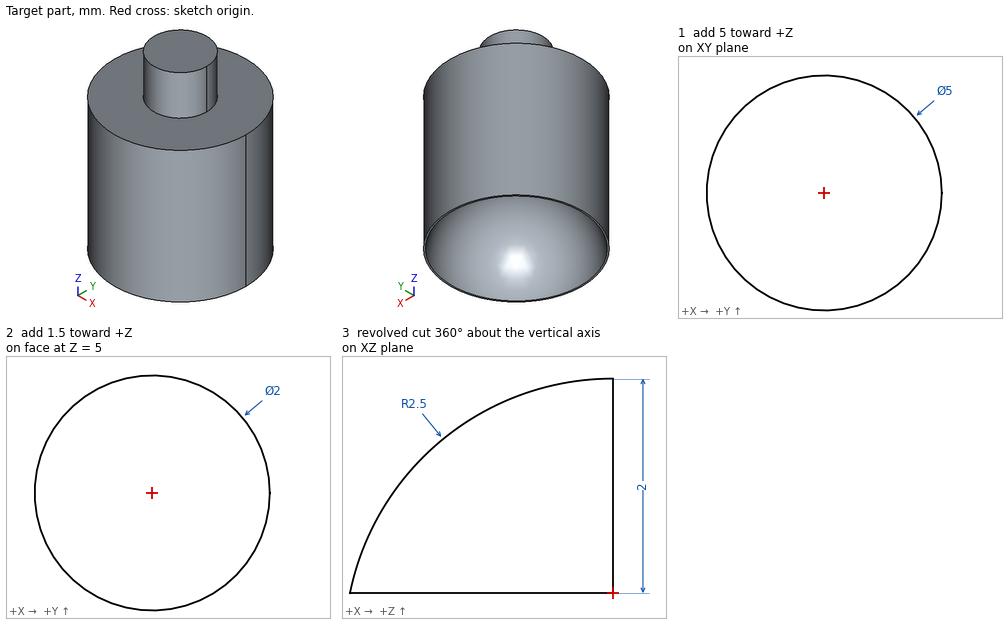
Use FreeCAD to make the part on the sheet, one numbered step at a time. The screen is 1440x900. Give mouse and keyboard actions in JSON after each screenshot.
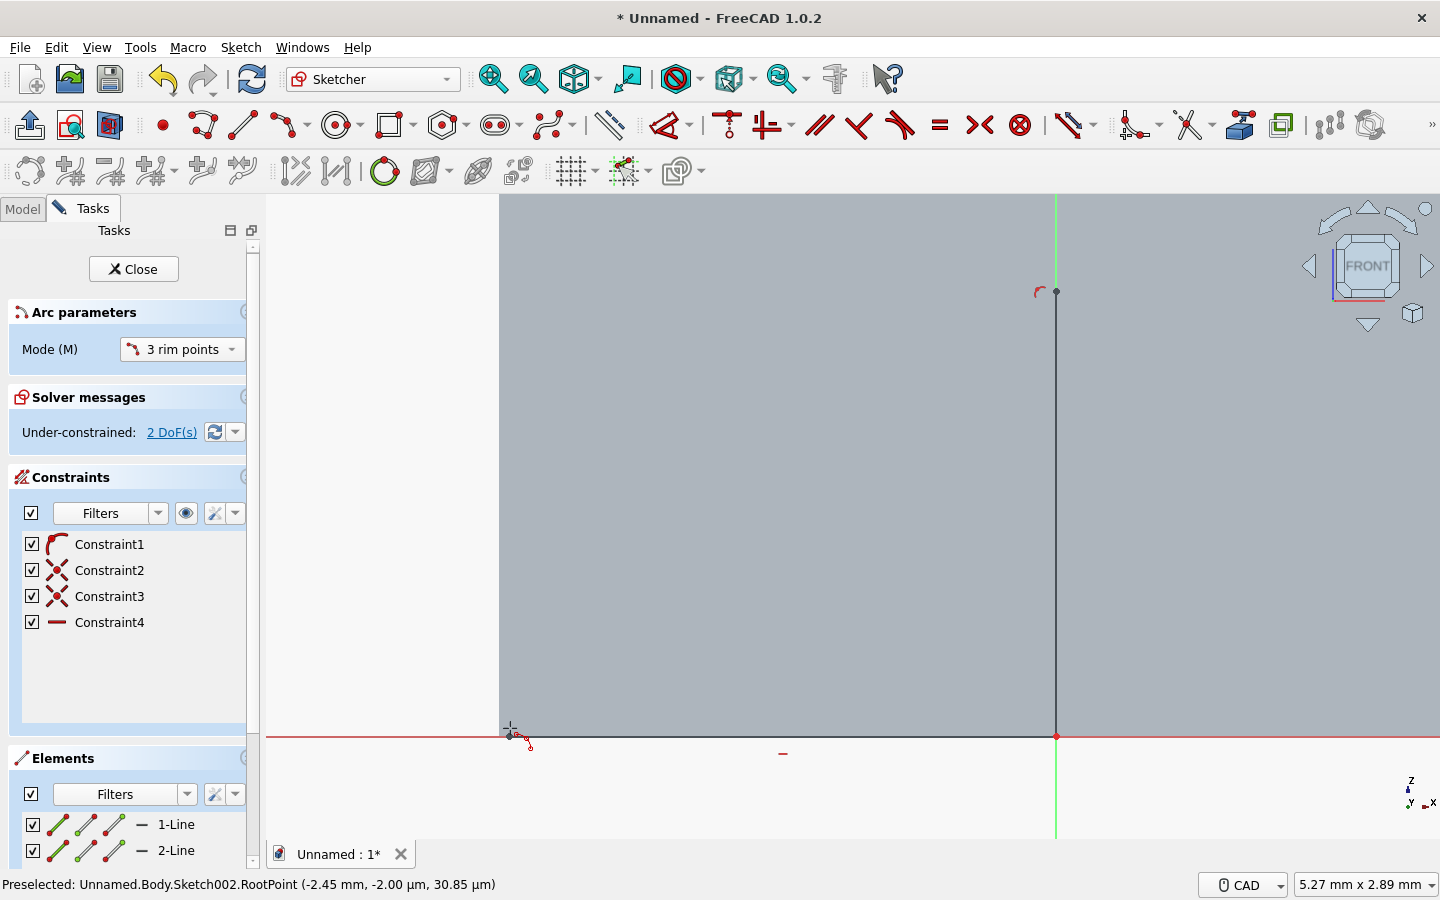
{"action": "left_click", "coordinate": [510, 737]}
{"action": "left_click", "coordinate": [1056, 292]}
{"action": "left_click", "coordinate": [704, 417]}
{"action": "key", "text": "Escape"}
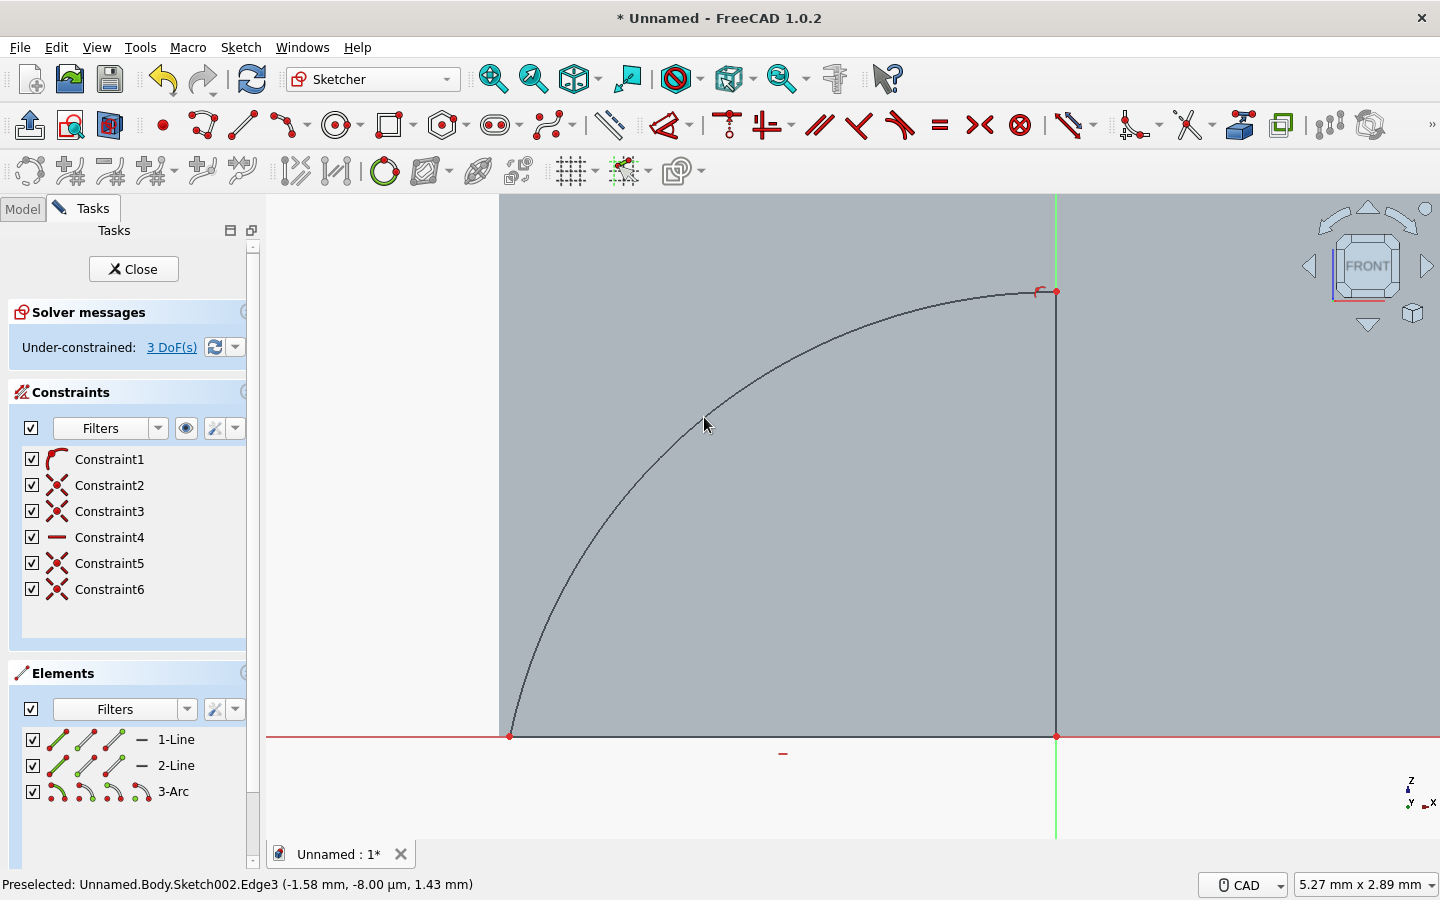
{"action": "scroll", "coordinate": [787, 269], "scroll_direction": "down", "scroll_amount": 1}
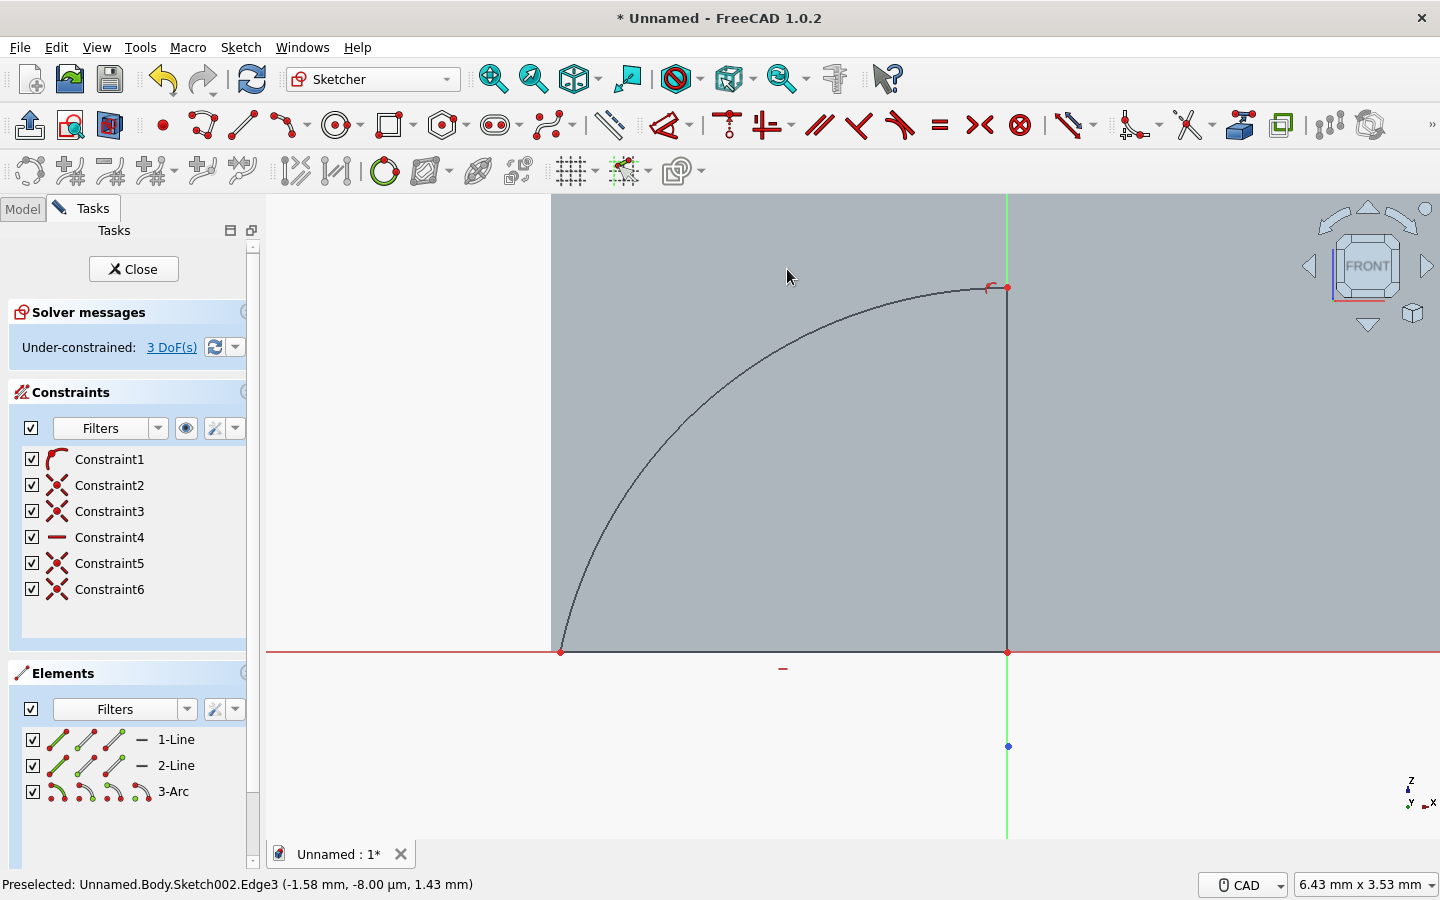
{"action": "left_click", "coordinate": [1009, 746]}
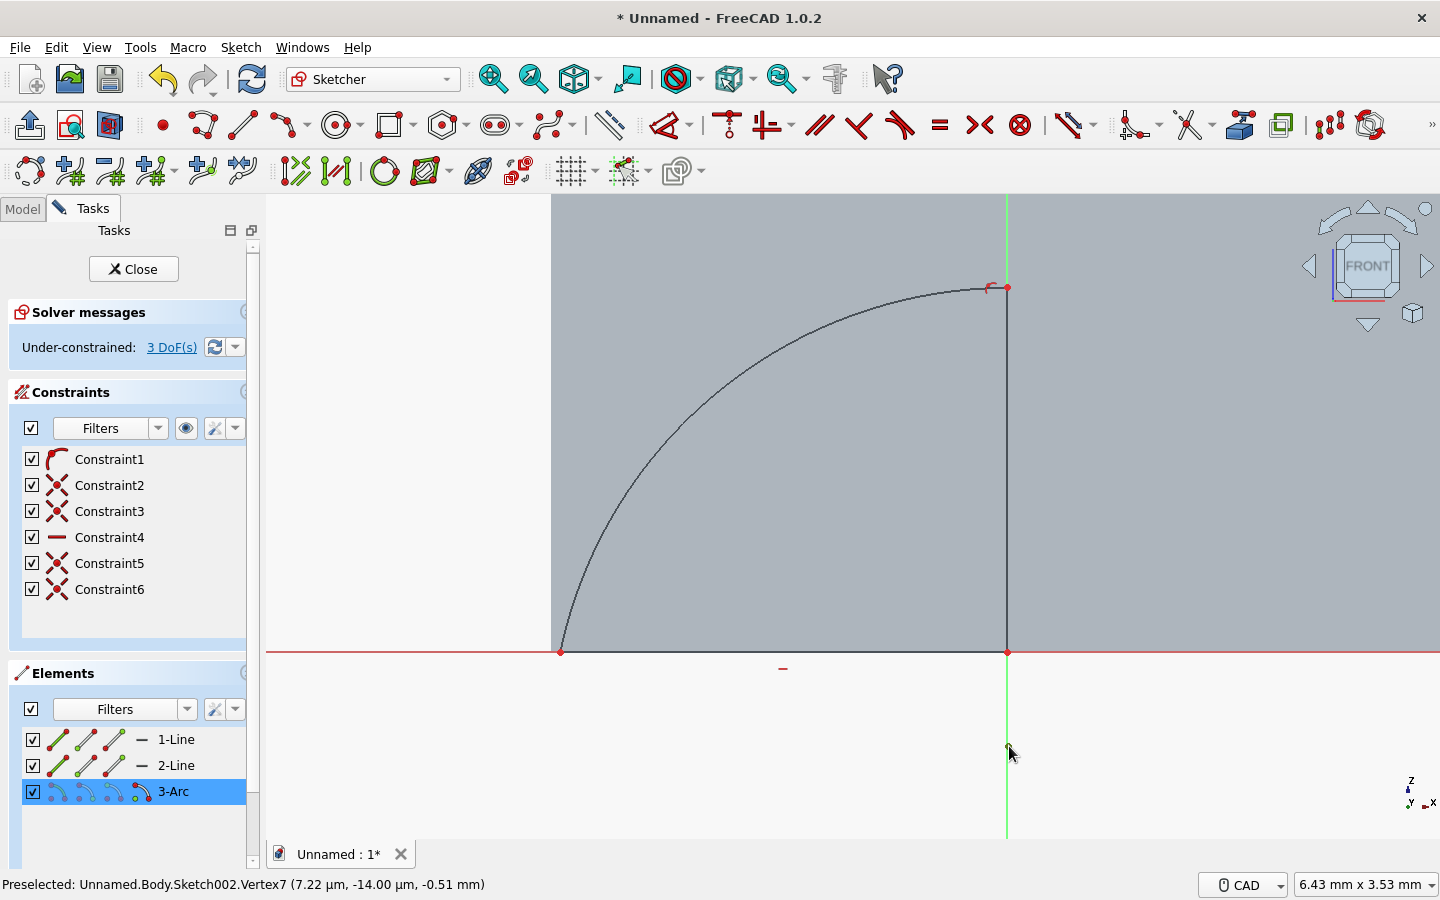
{"action": "left_click", "coordinate": [1007, 769]}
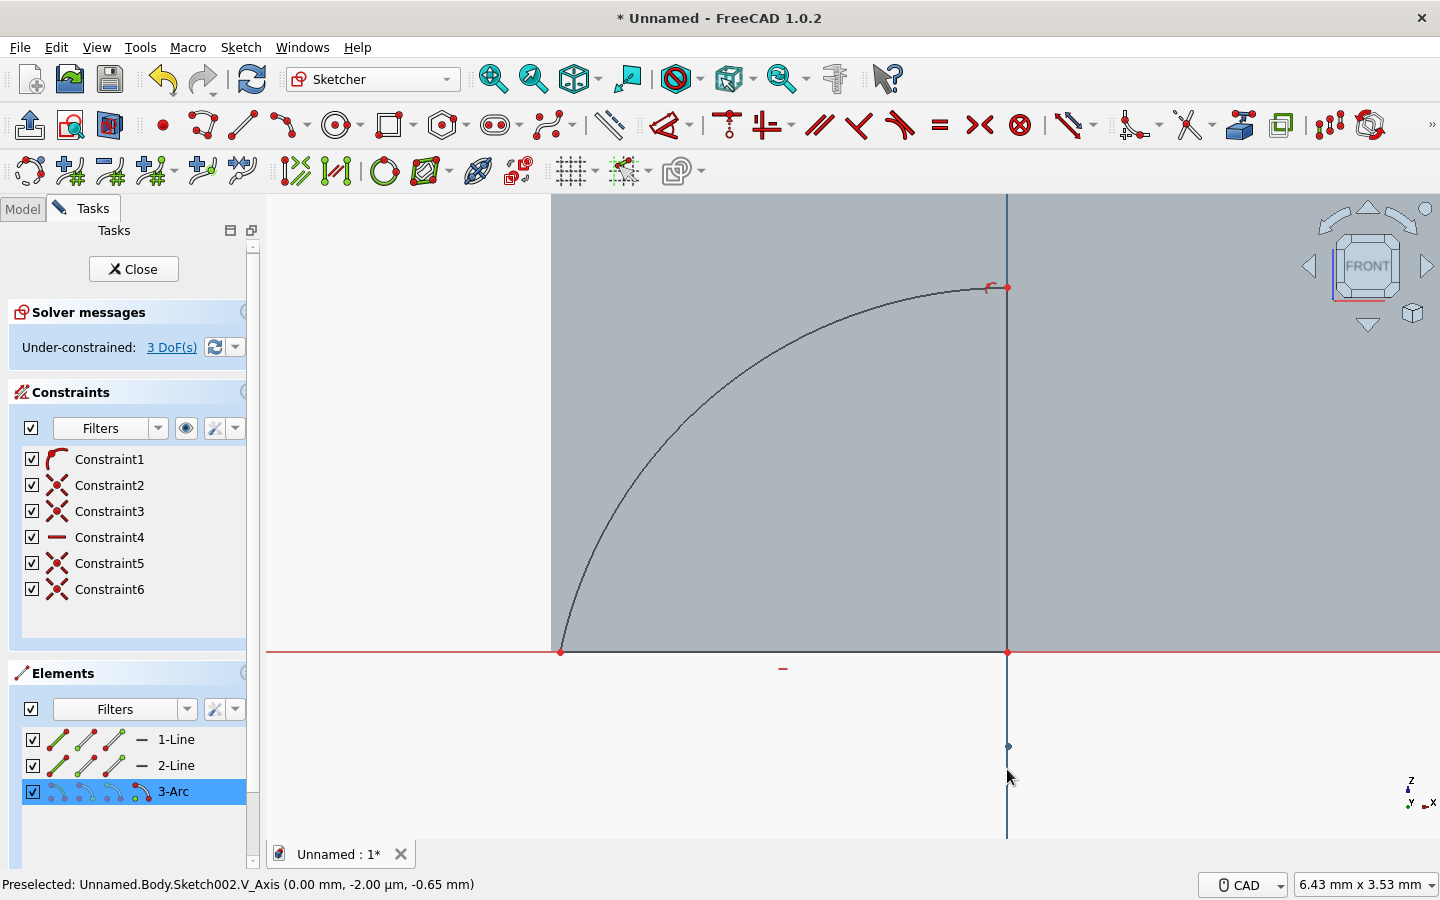
{"action": "left_click", "coordinate": [728, 126]}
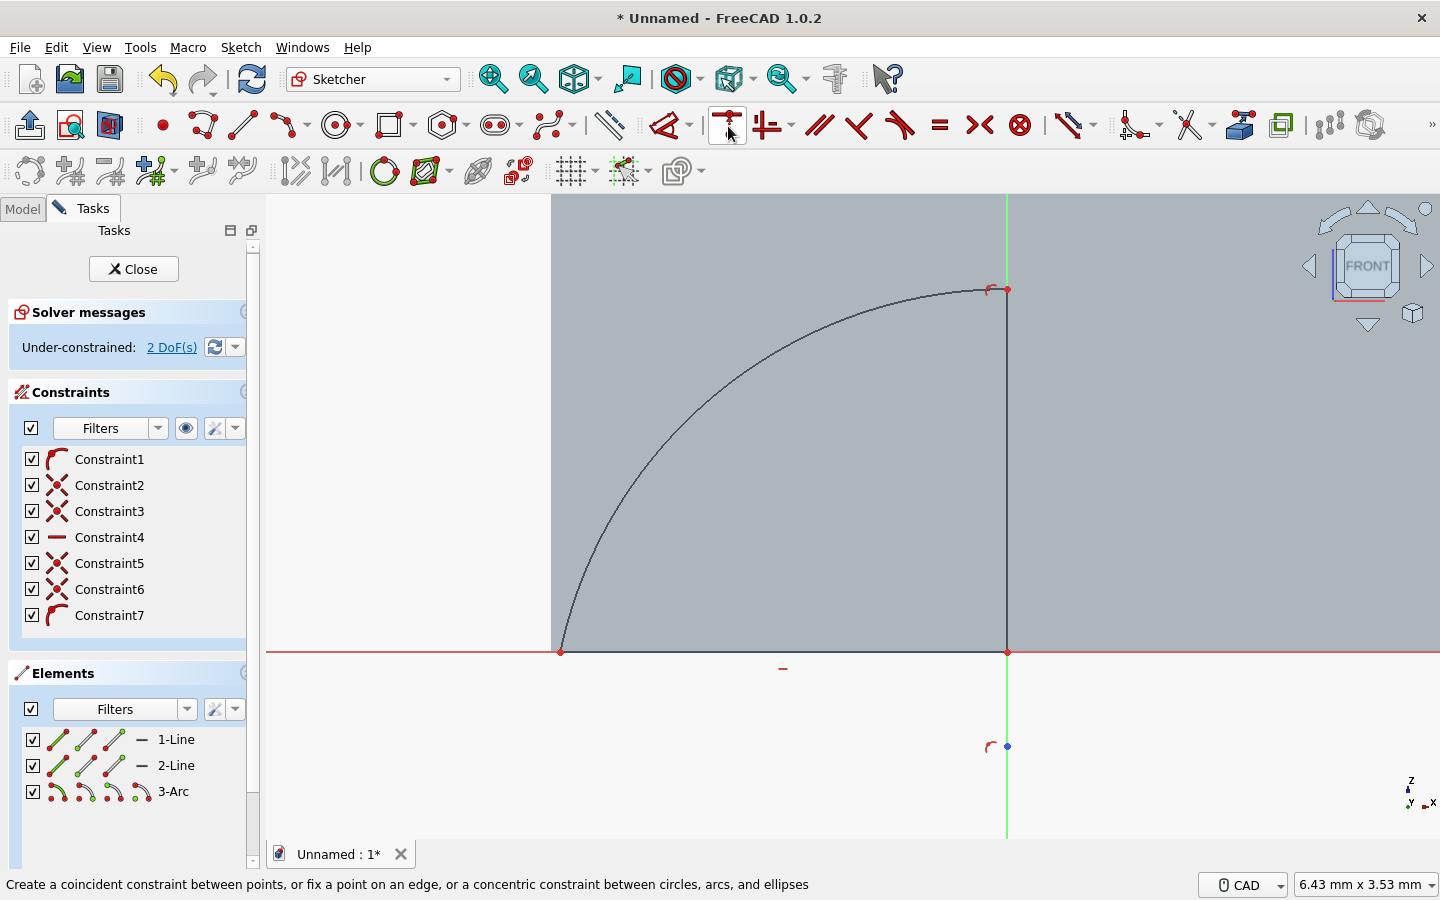
{"action": "left_click", "coordinate": [664, 126]}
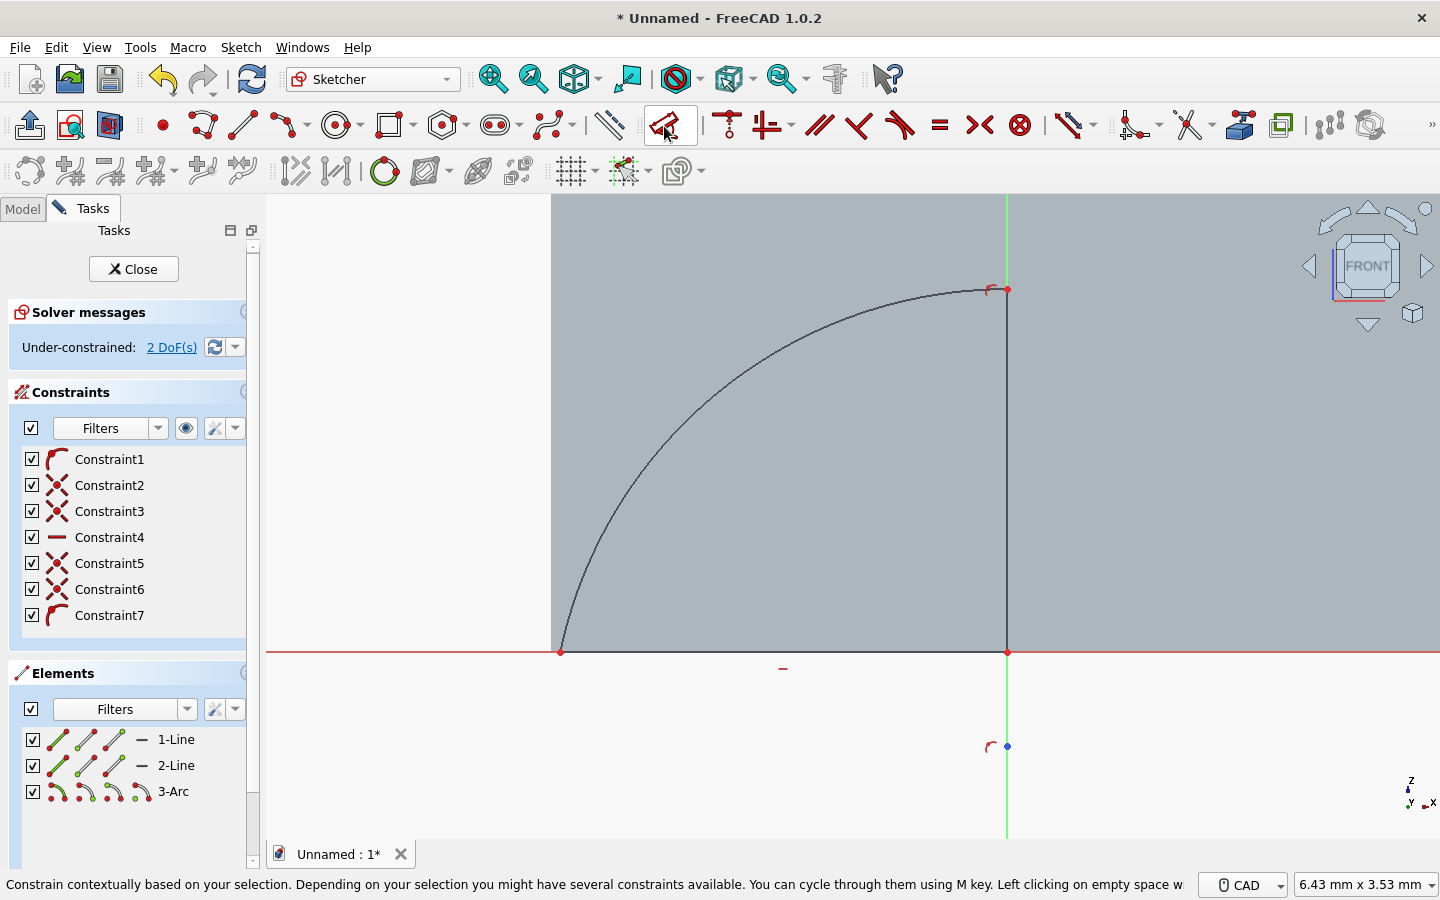
{"action": "left_click", "coordinate": [826, 327]}
{"action": "left_click", "coordinate": [813, 298]}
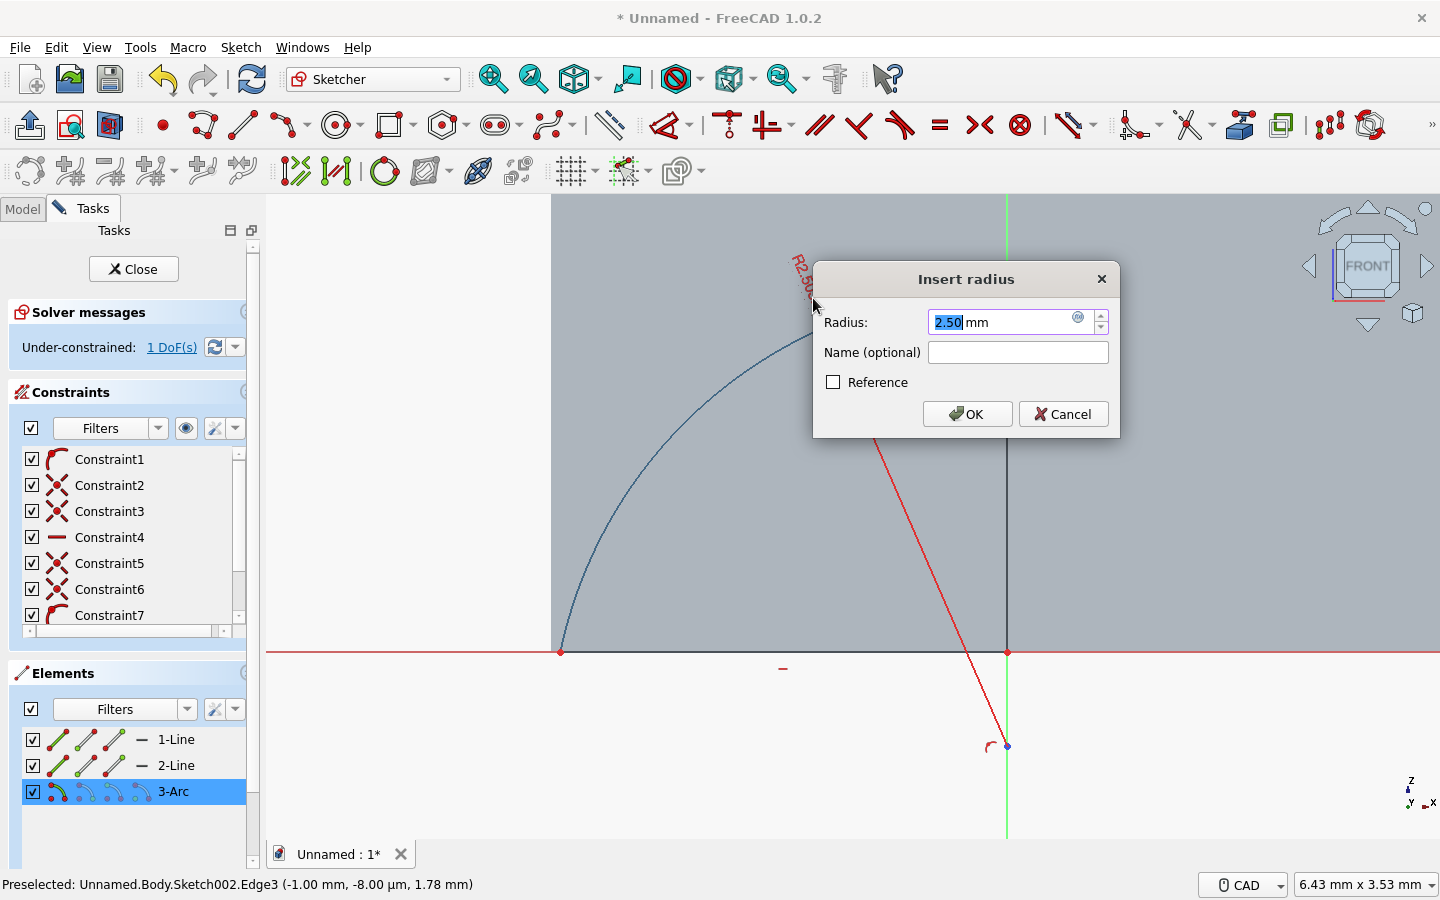
{"action": "type", "text": "2.5"}
{"action": "key", "text": "Return"}